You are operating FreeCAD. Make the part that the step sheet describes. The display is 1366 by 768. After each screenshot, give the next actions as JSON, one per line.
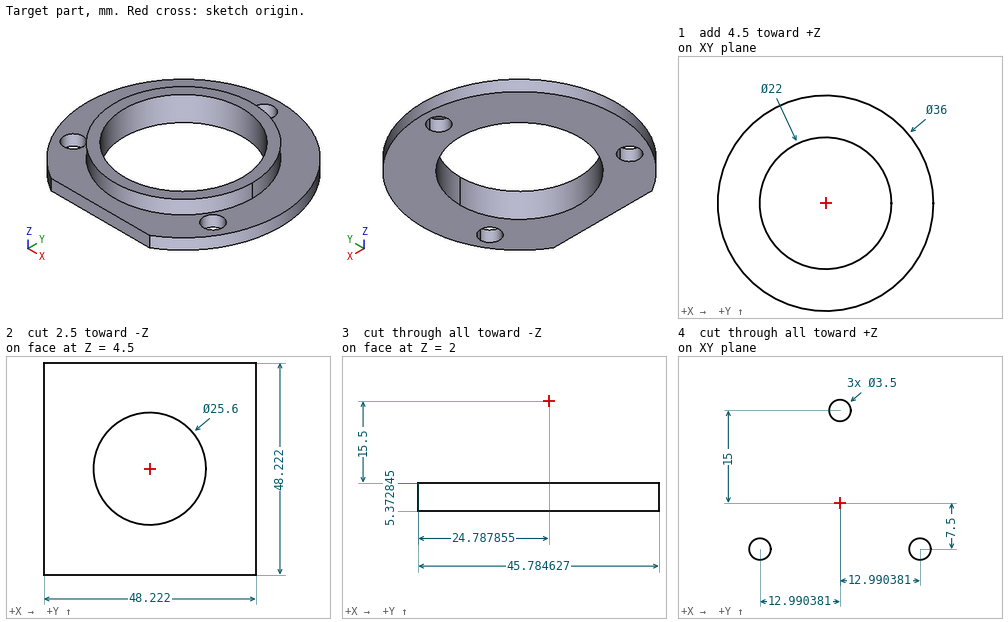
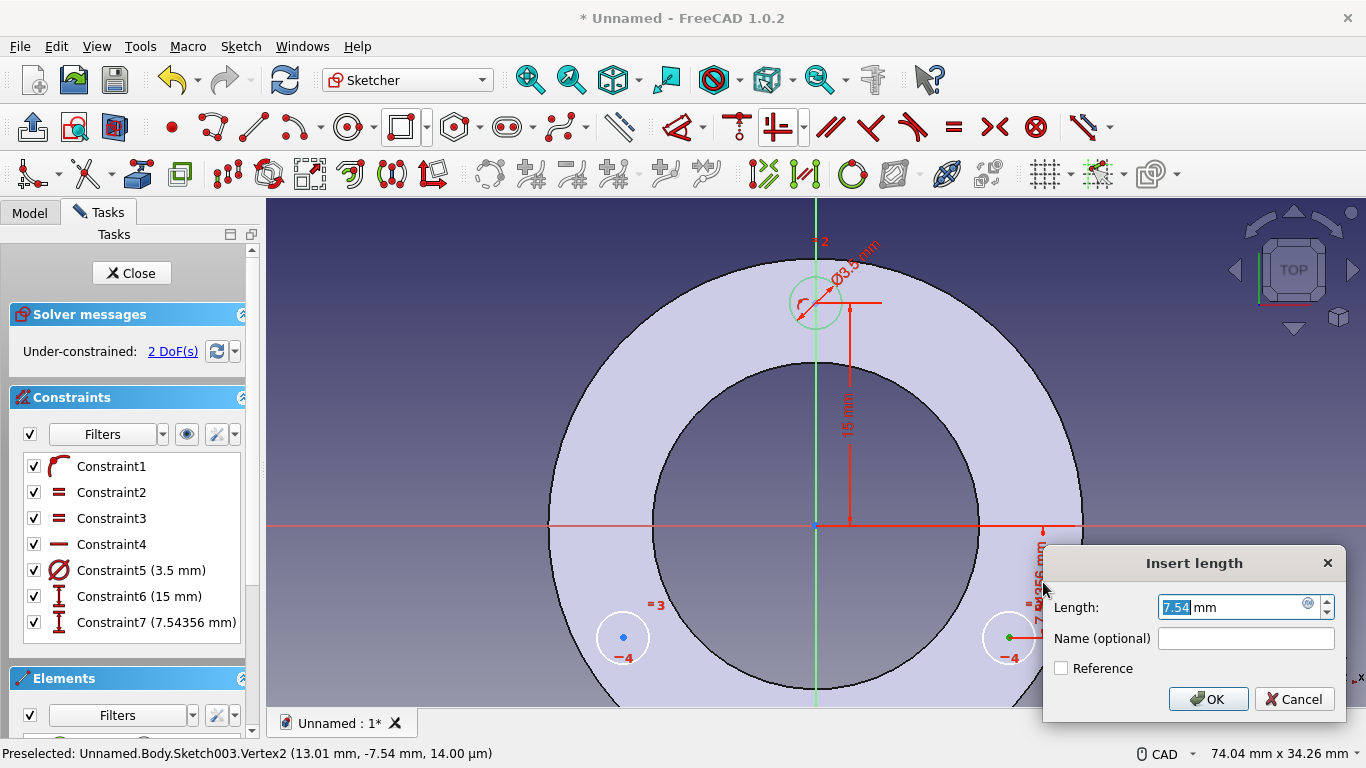
{"action": "type", "text": "7.5"}
{"action": "key", "text": "Return"}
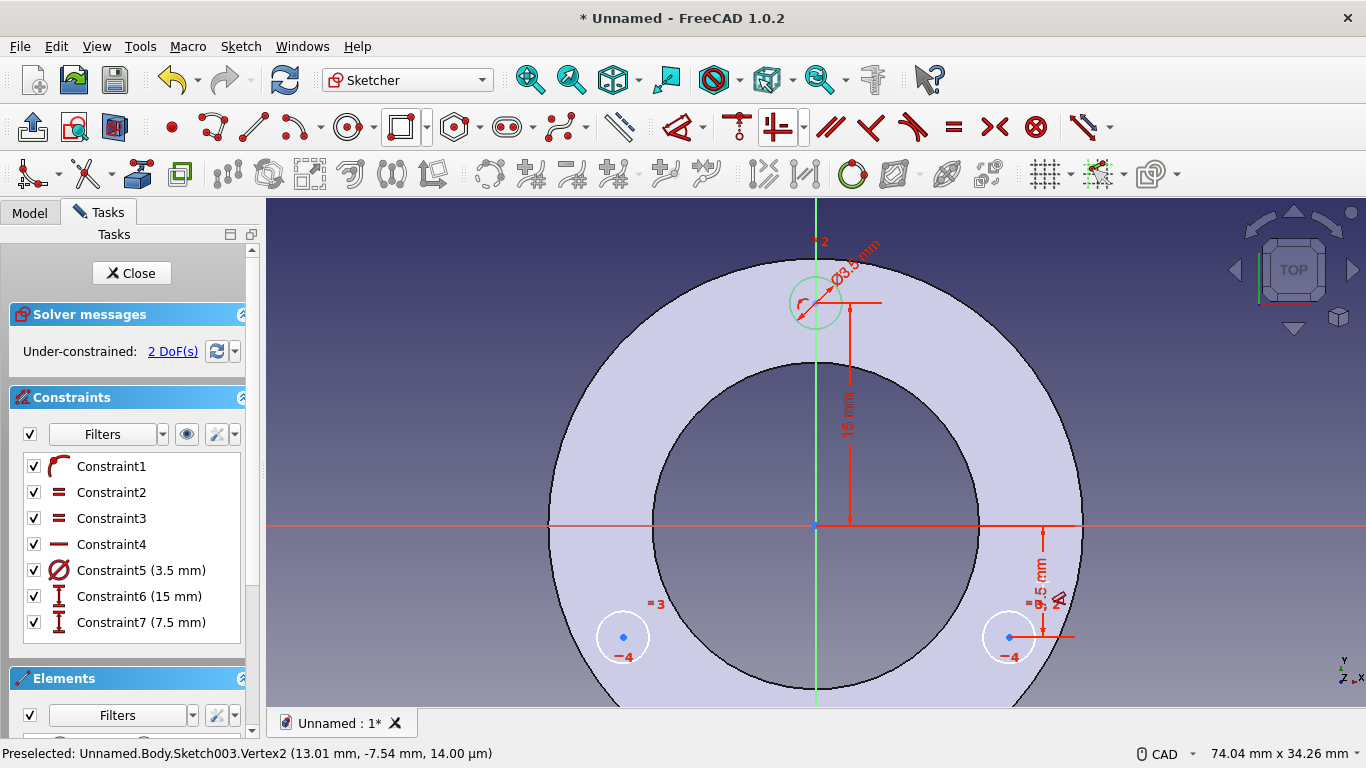
{"action": "left_click", "coordinate": [1009, 637]}
{"action": "left_click", "coordinate": [912, 671]}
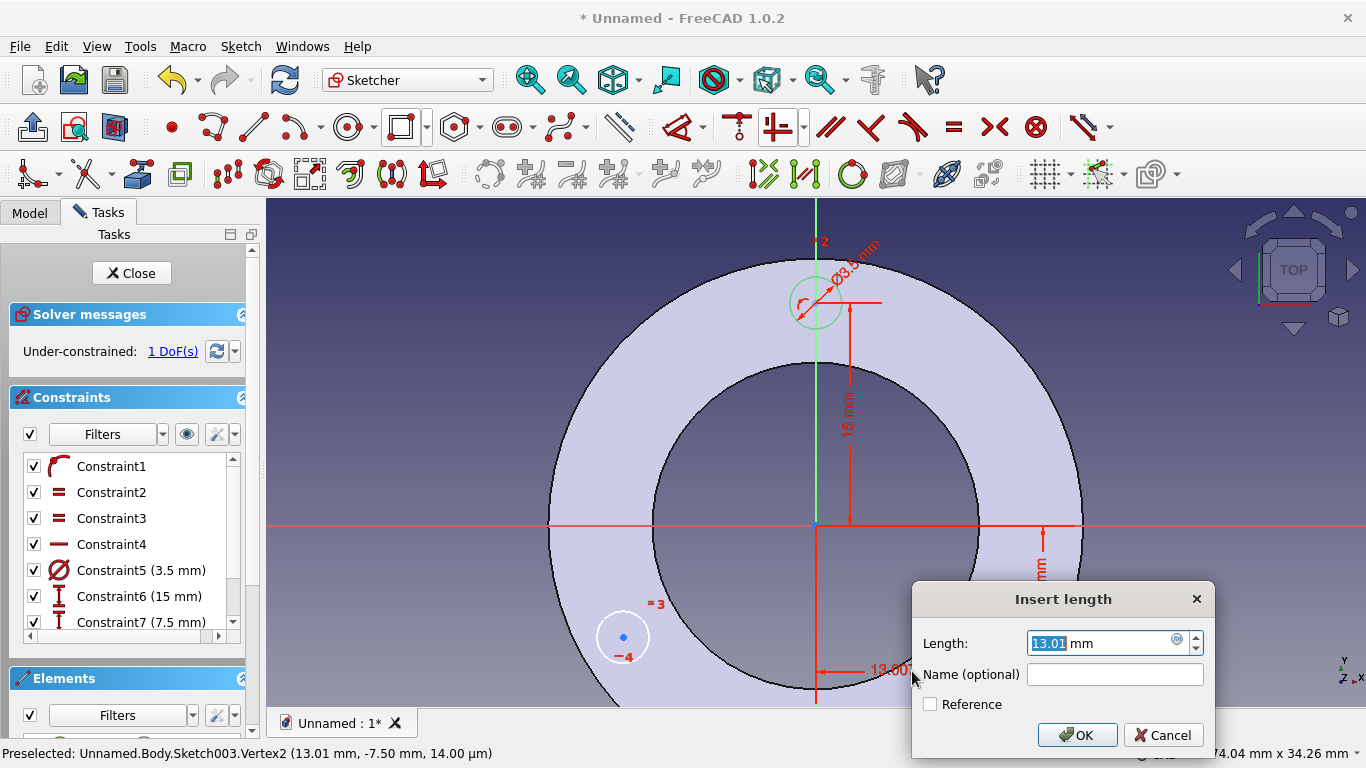
{"action": "type", "text": "12.990381"}
{"action": "key", "text": "Return"}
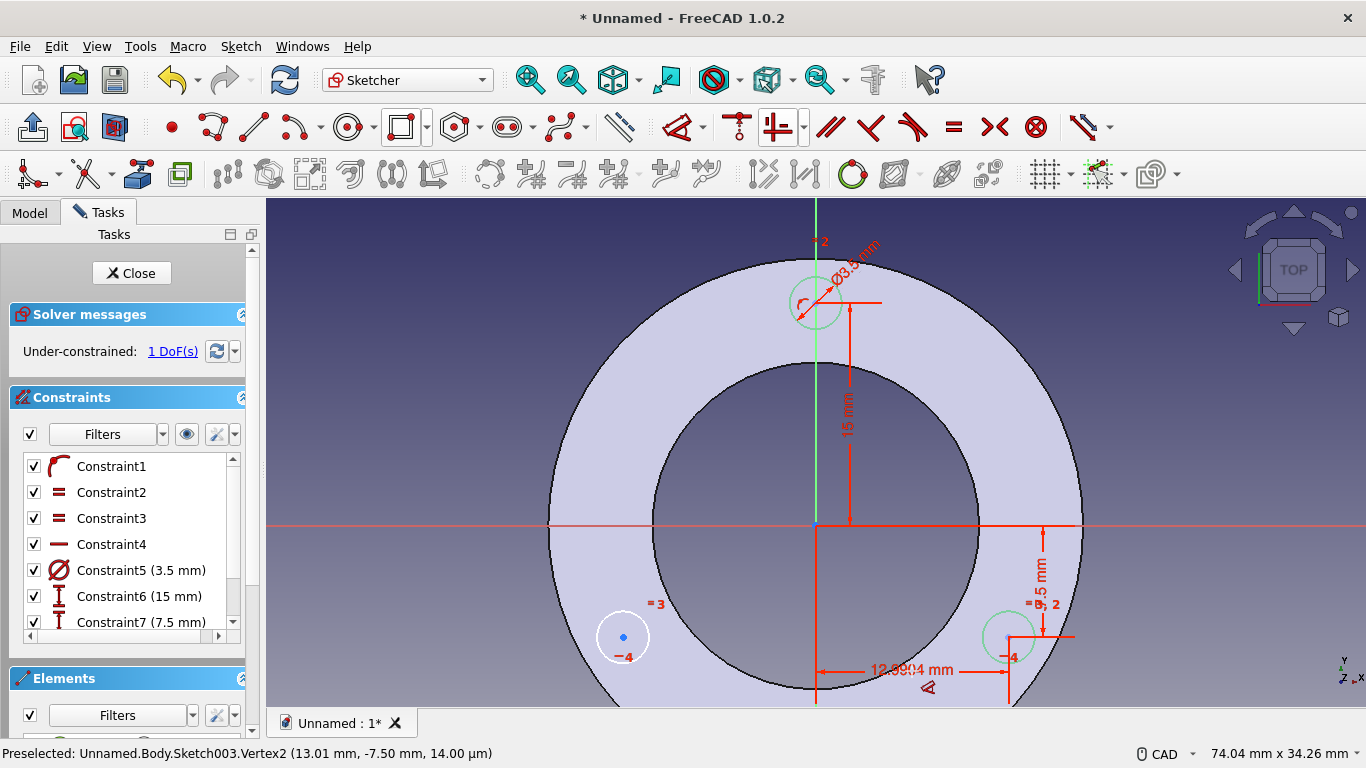
{"action": "left_click", "coordinate": [623, 637]}
{"action": "left_click", "coordinate": [719, 671]}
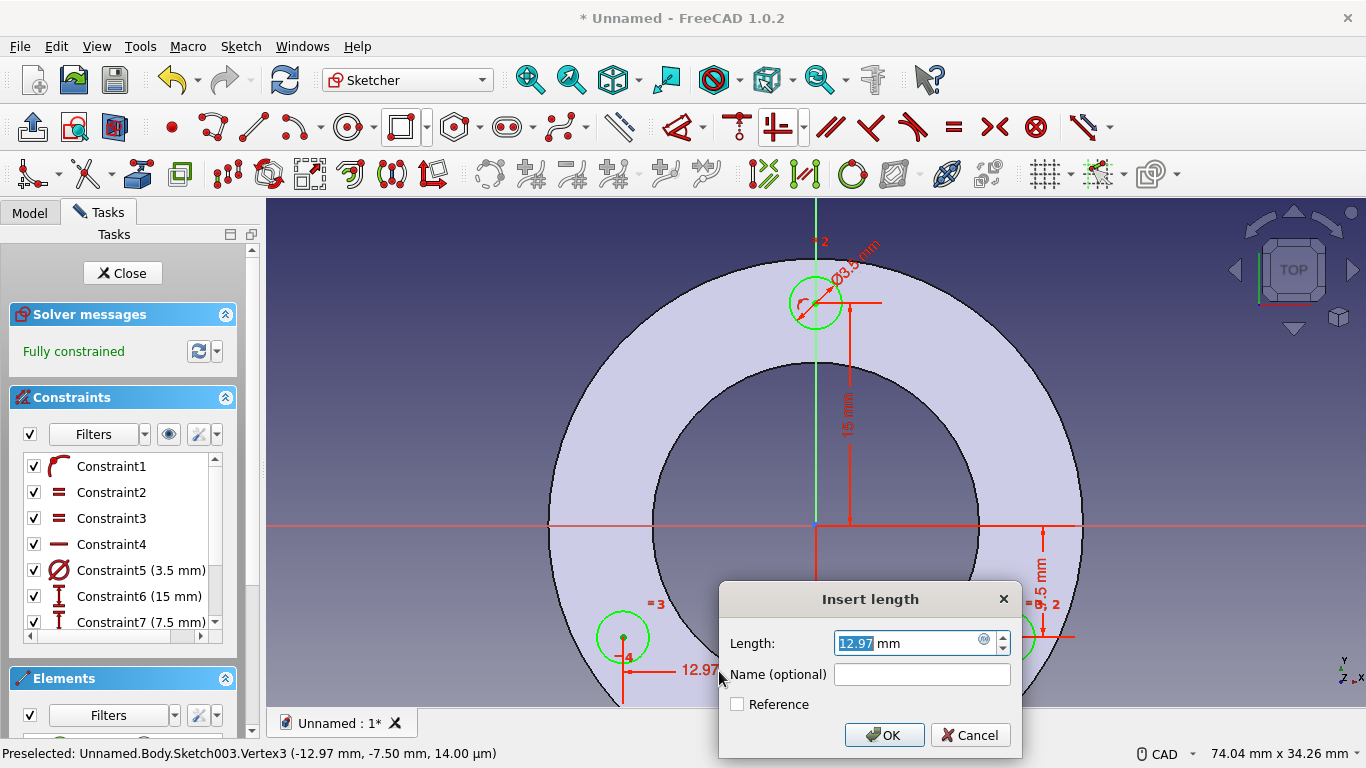
{"action": "type", "text": "12.990381"}
{"action": "key", "text": "Return"}
{"action": "key", "text": "Escape"}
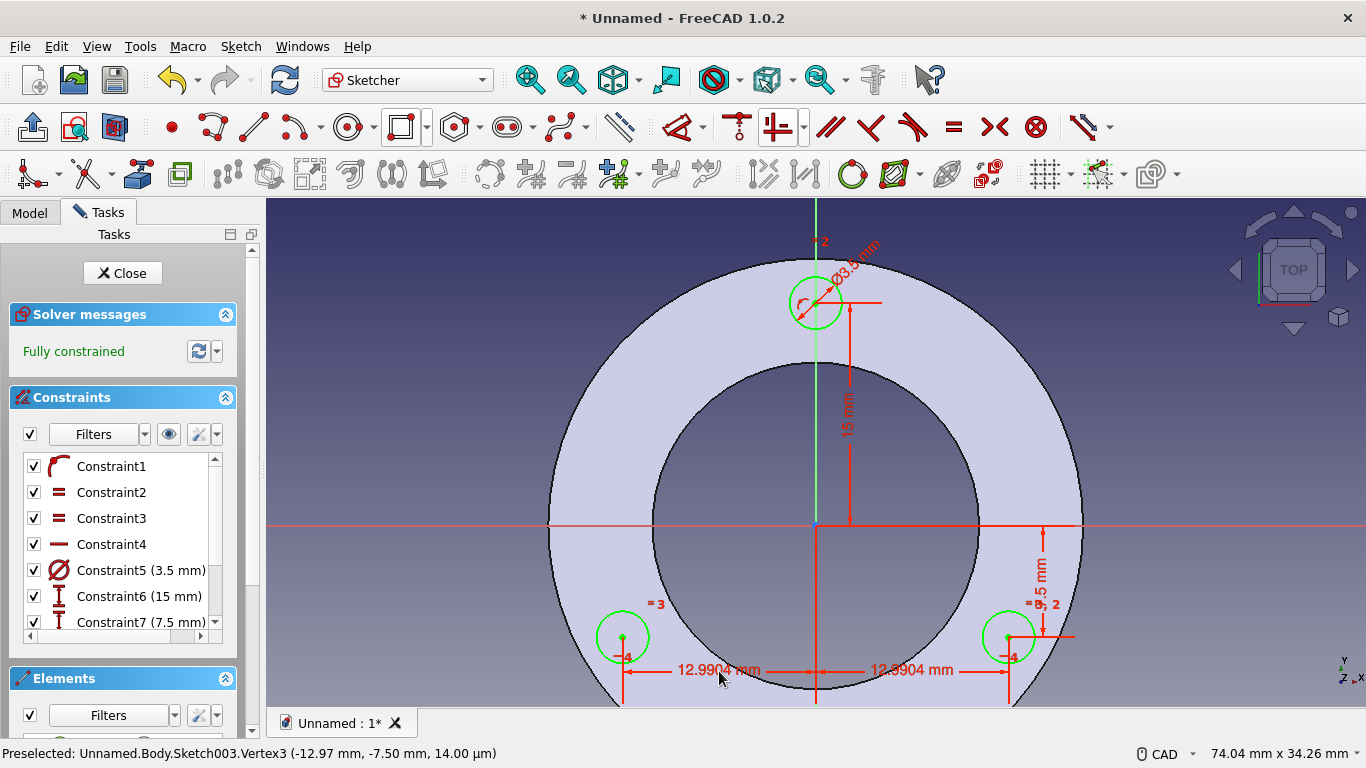
{"action": "left_click", "coordinate": [123, 273]}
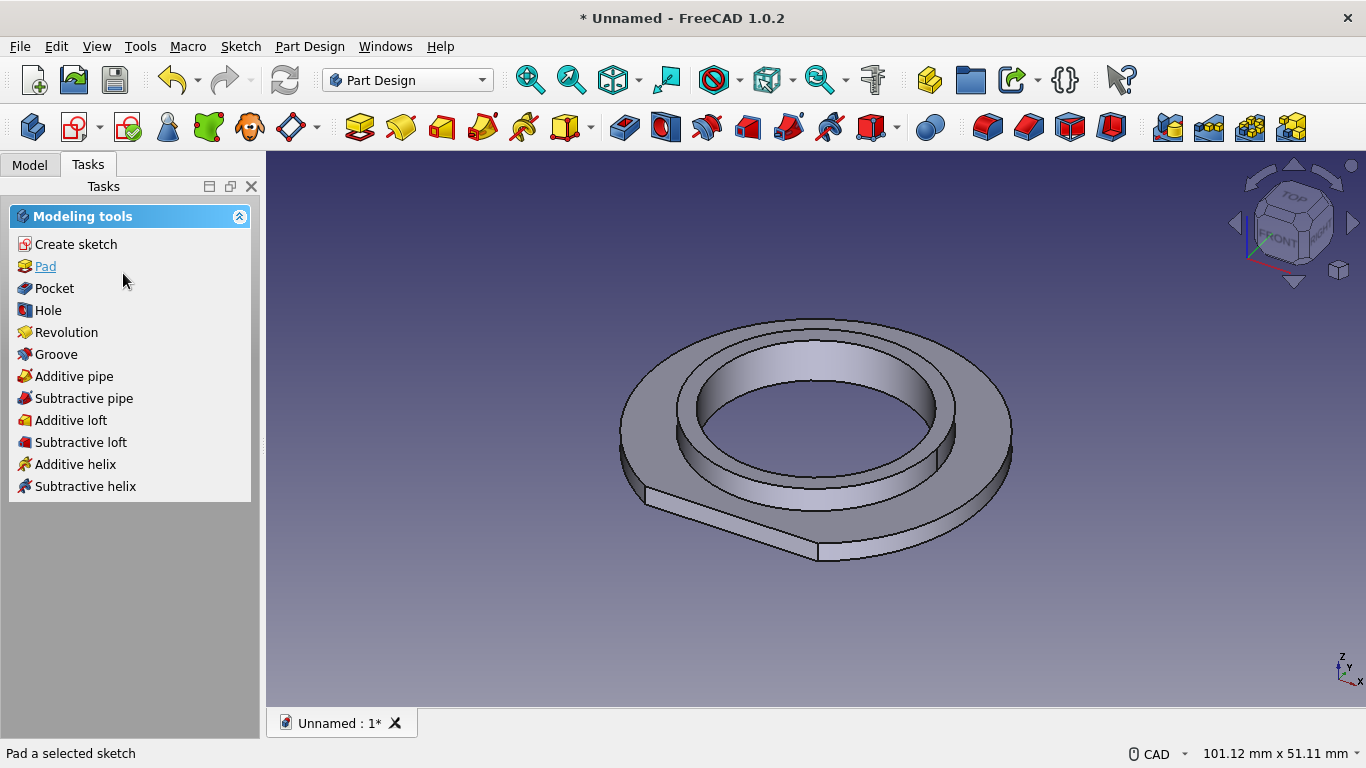
{"action": "left_click", "coordinate": [625, 128]}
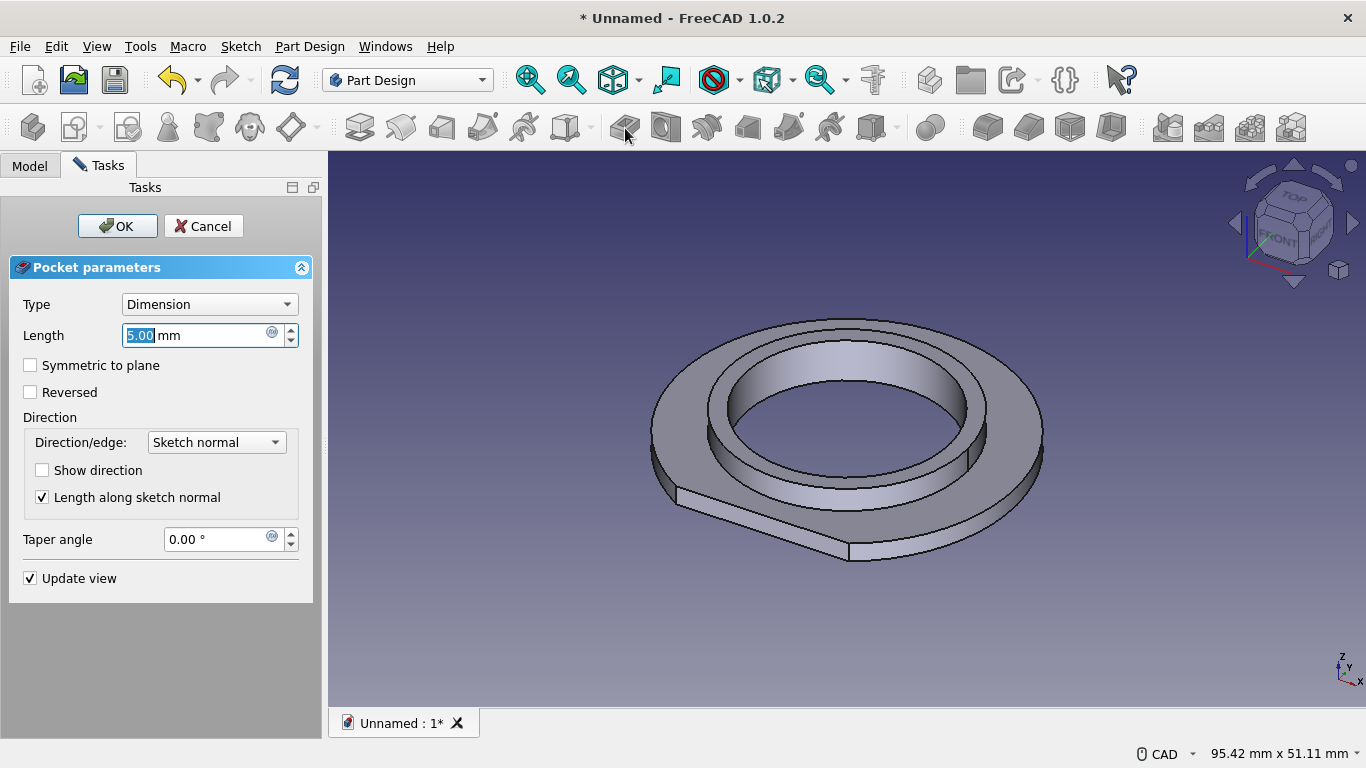
{"action": "left_click", "coordinate": [210, 304]}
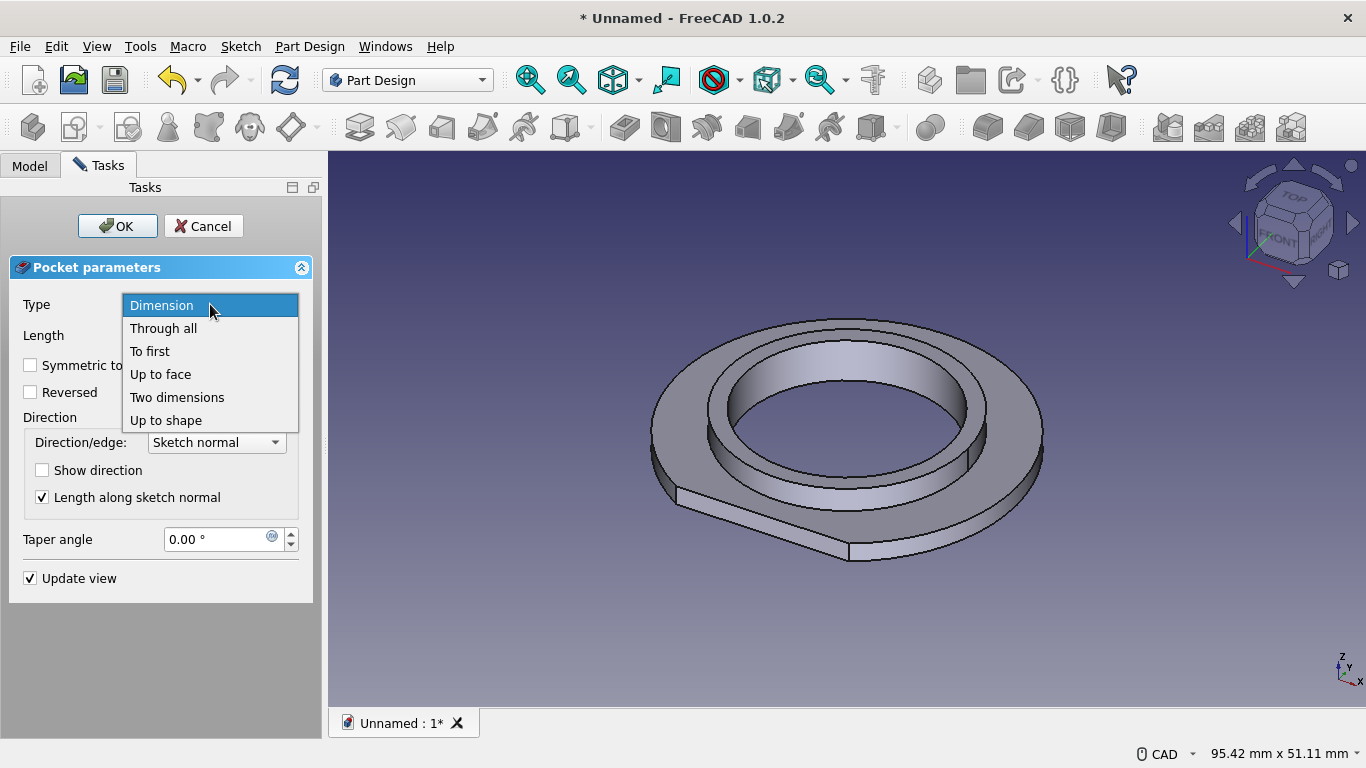
{"action": "left_click", "coordinate": [208, 328]}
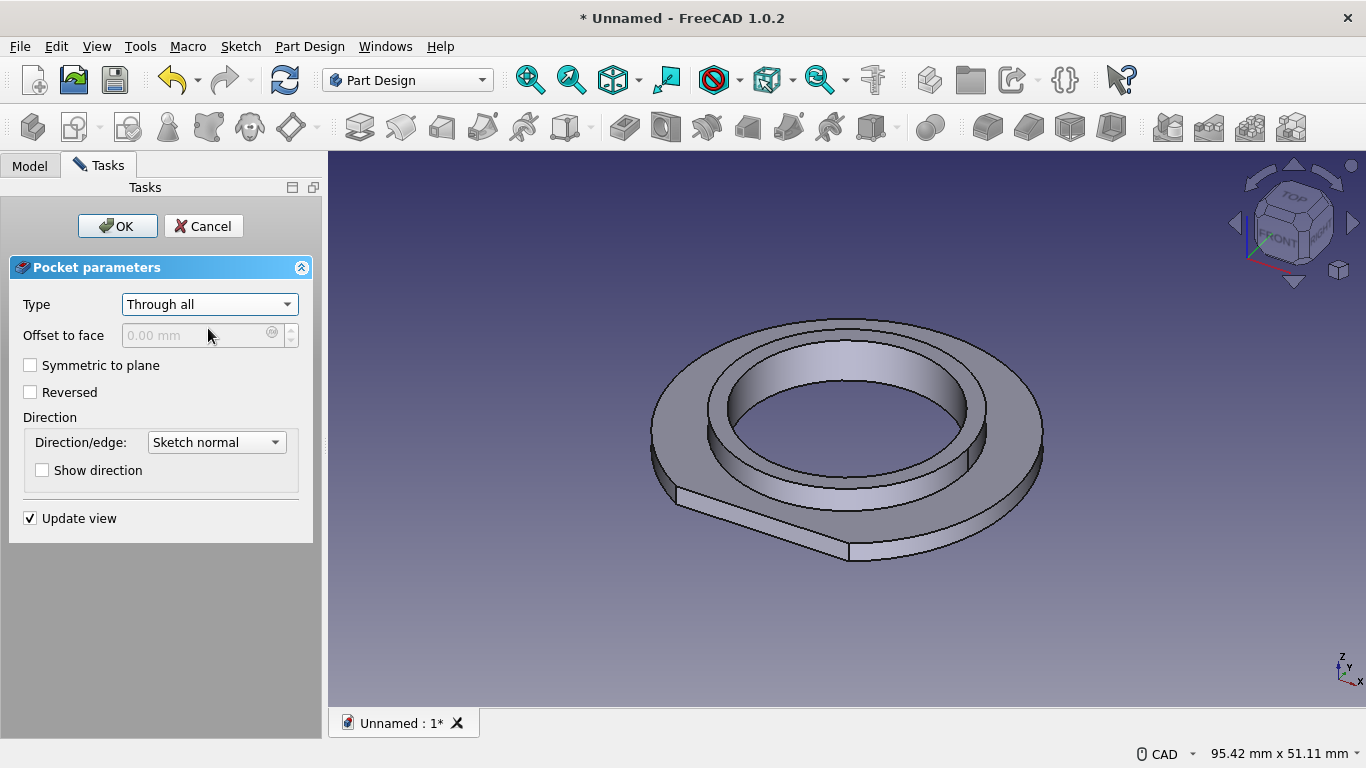
{"action": "left_click", "coordinate": [31, 392]}